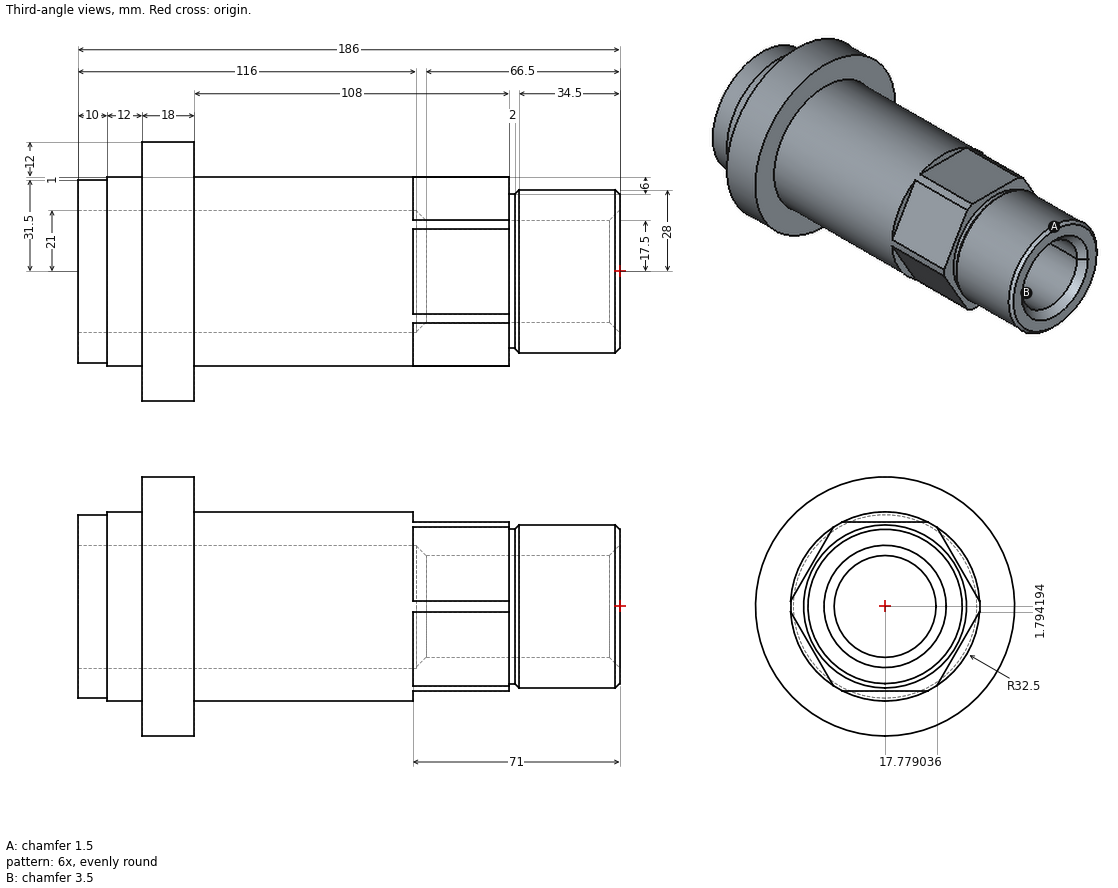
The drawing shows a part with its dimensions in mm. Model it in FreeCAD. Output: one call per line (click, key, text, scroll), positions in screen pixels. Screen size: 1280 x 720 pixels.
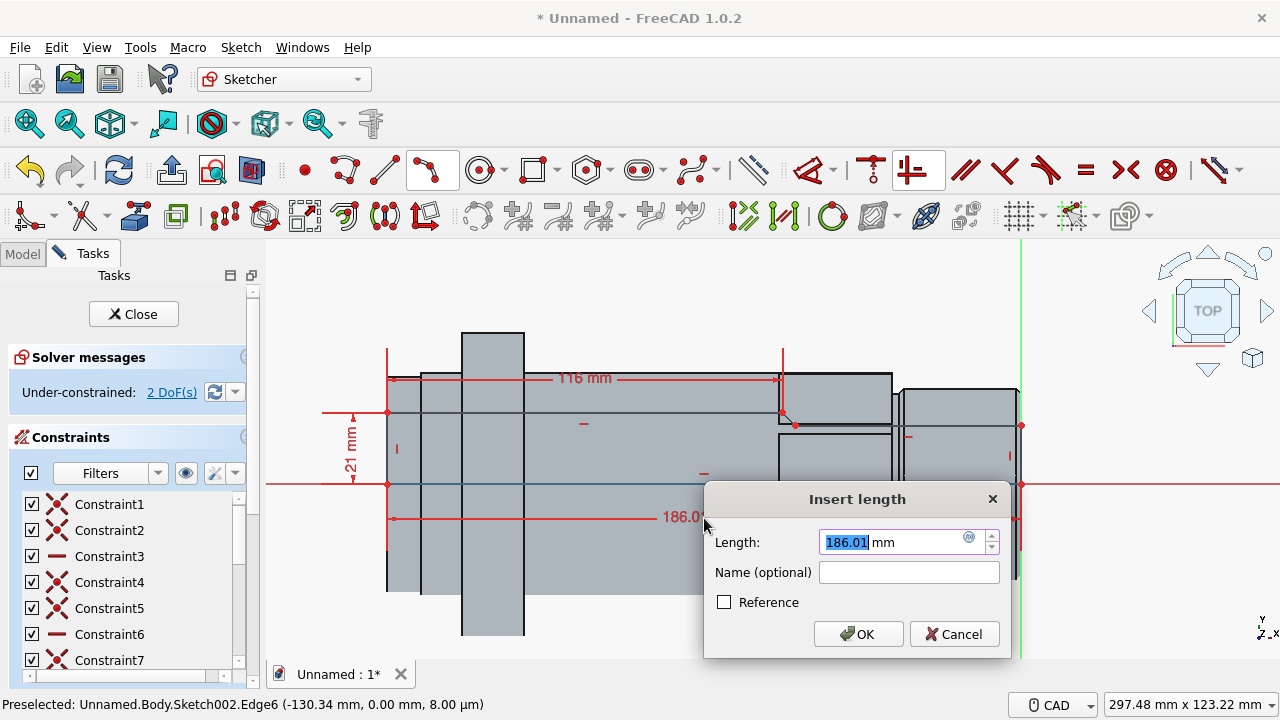
text(186)
key(Return)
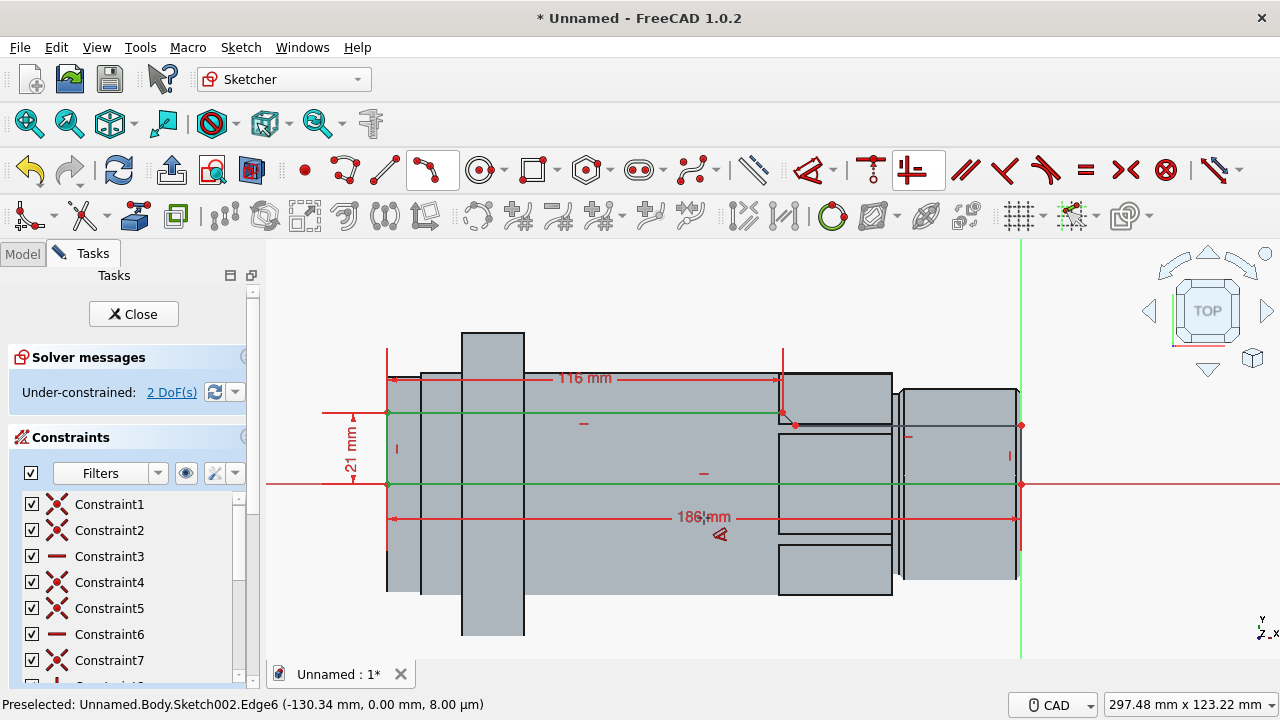
click(1021, 467)
click(1055, 455)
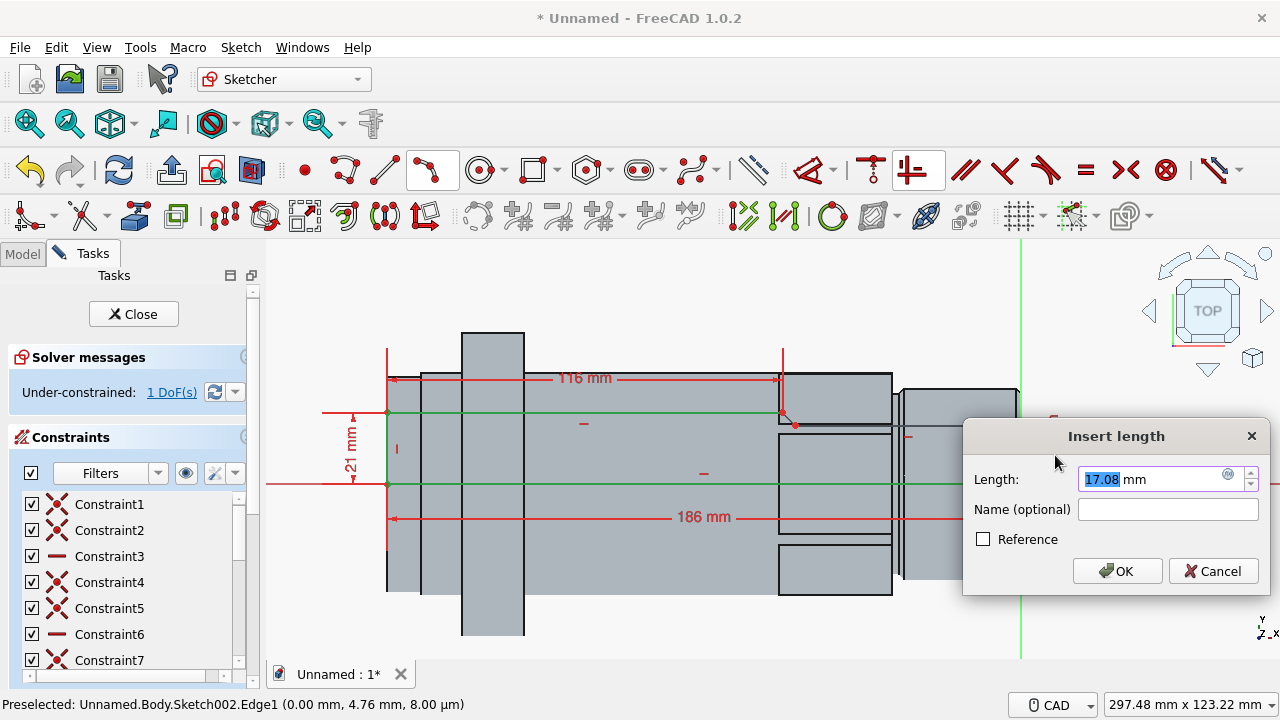
text(17.5)
key(Return)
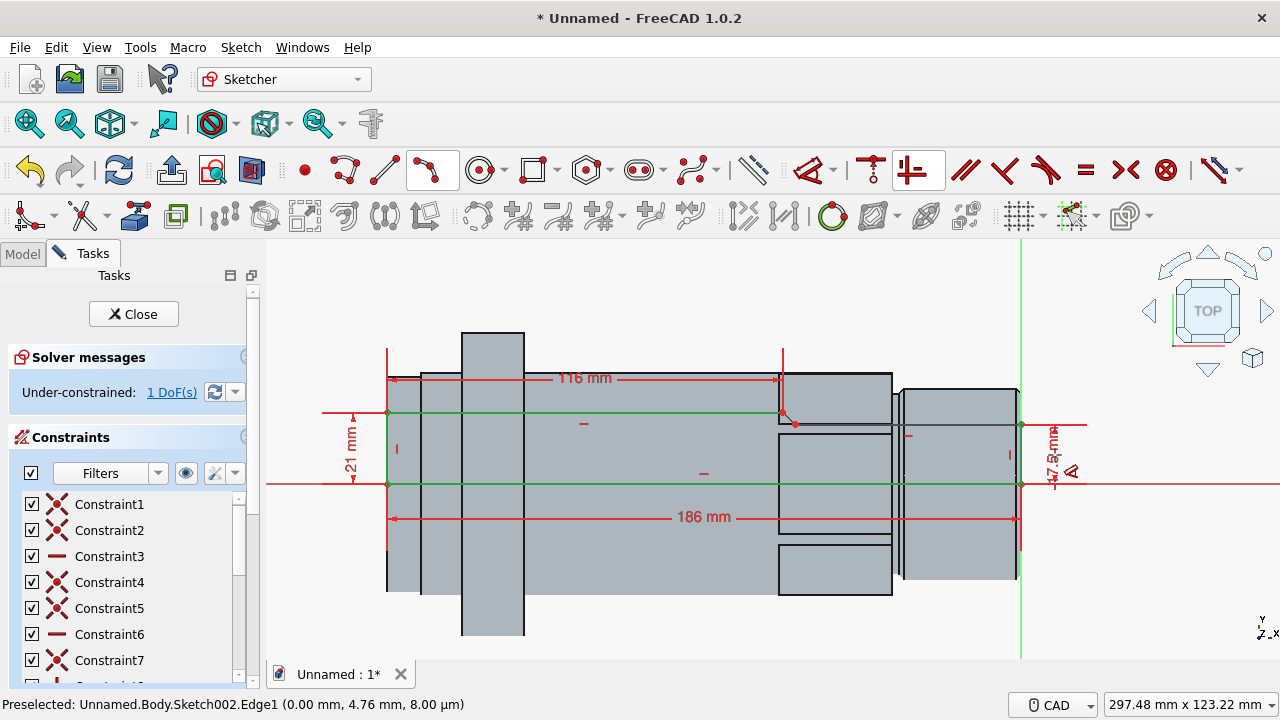
click(953, 425)
click(908, 391)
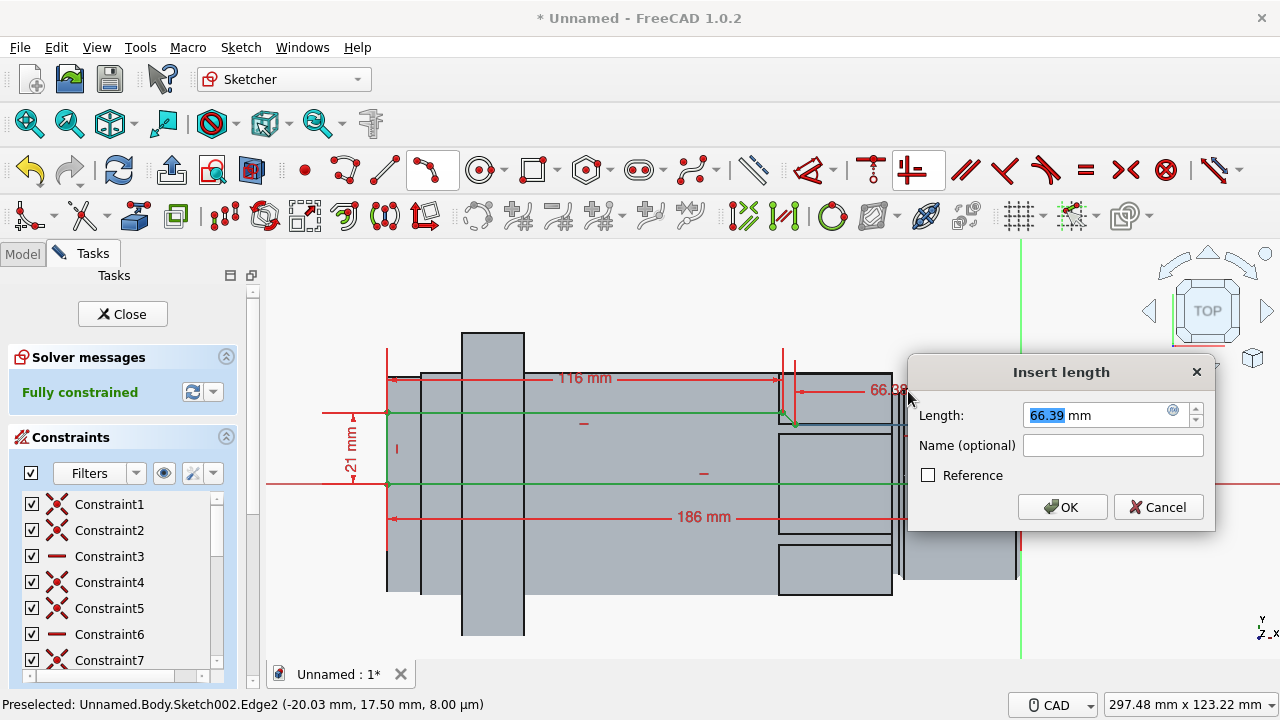
text(66.5)
key(Return)
key(Escape)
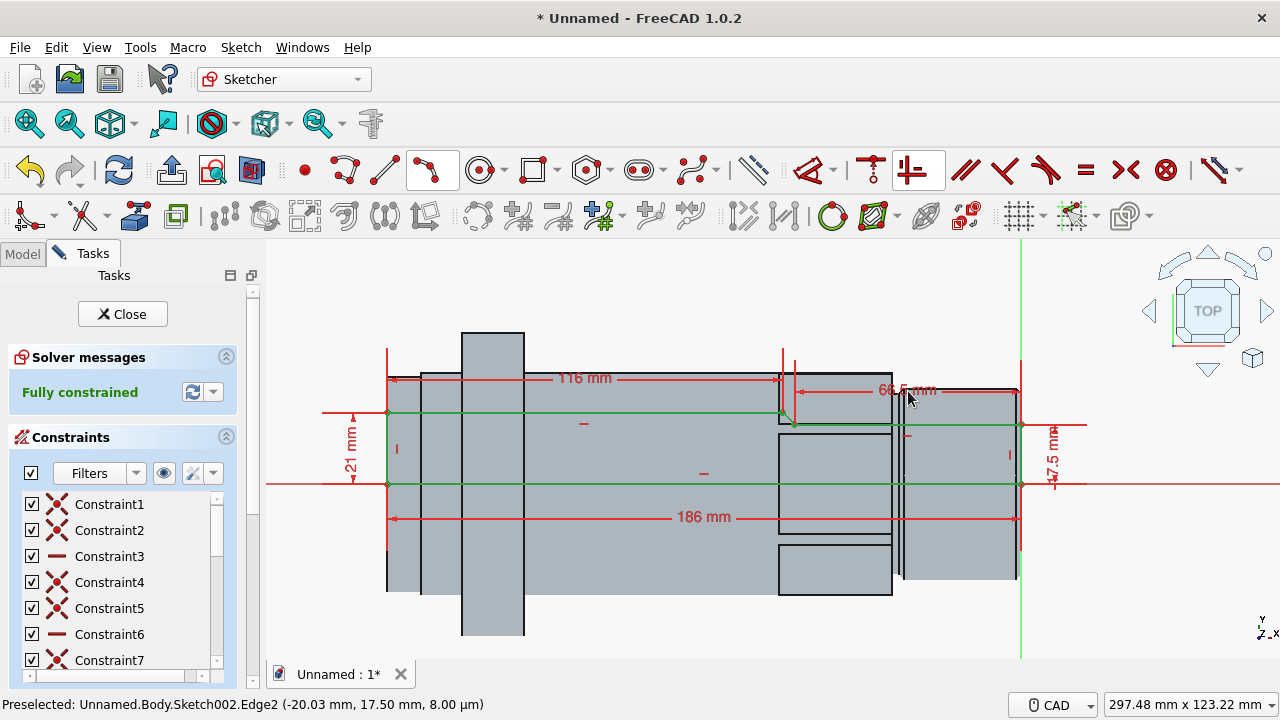
click(123, 314)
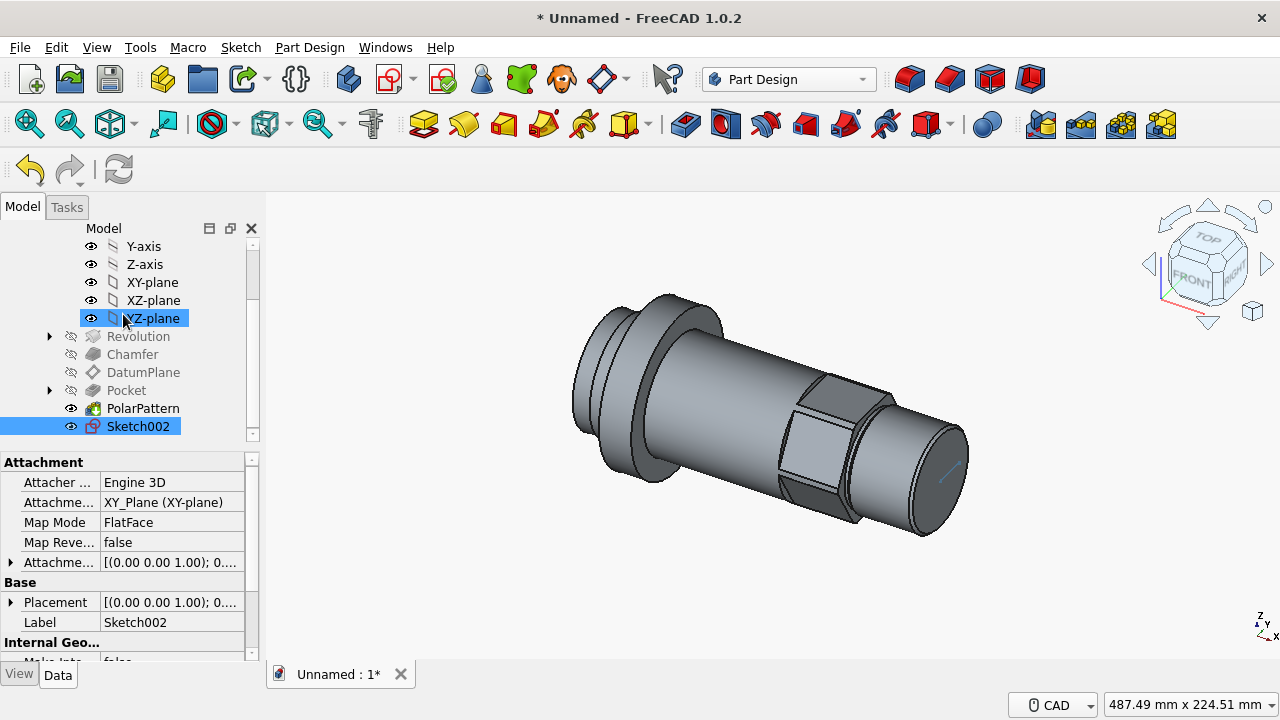
click(766, 124)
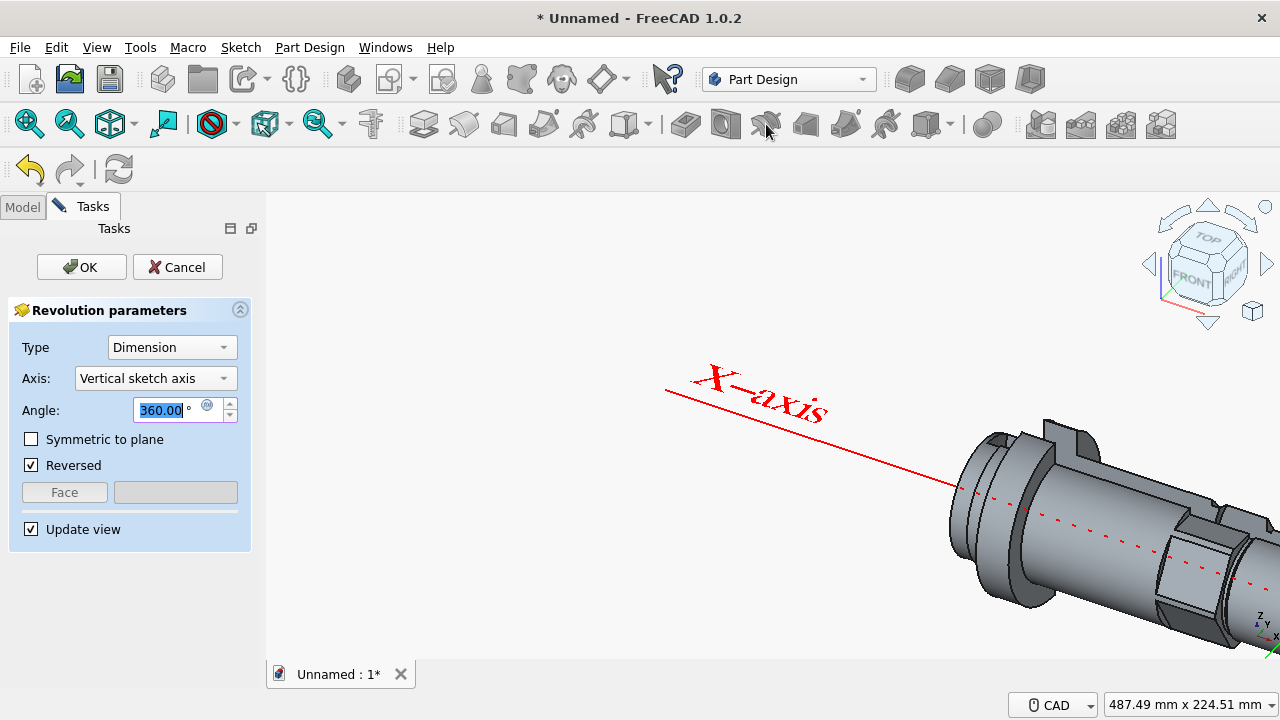
click(156, 378)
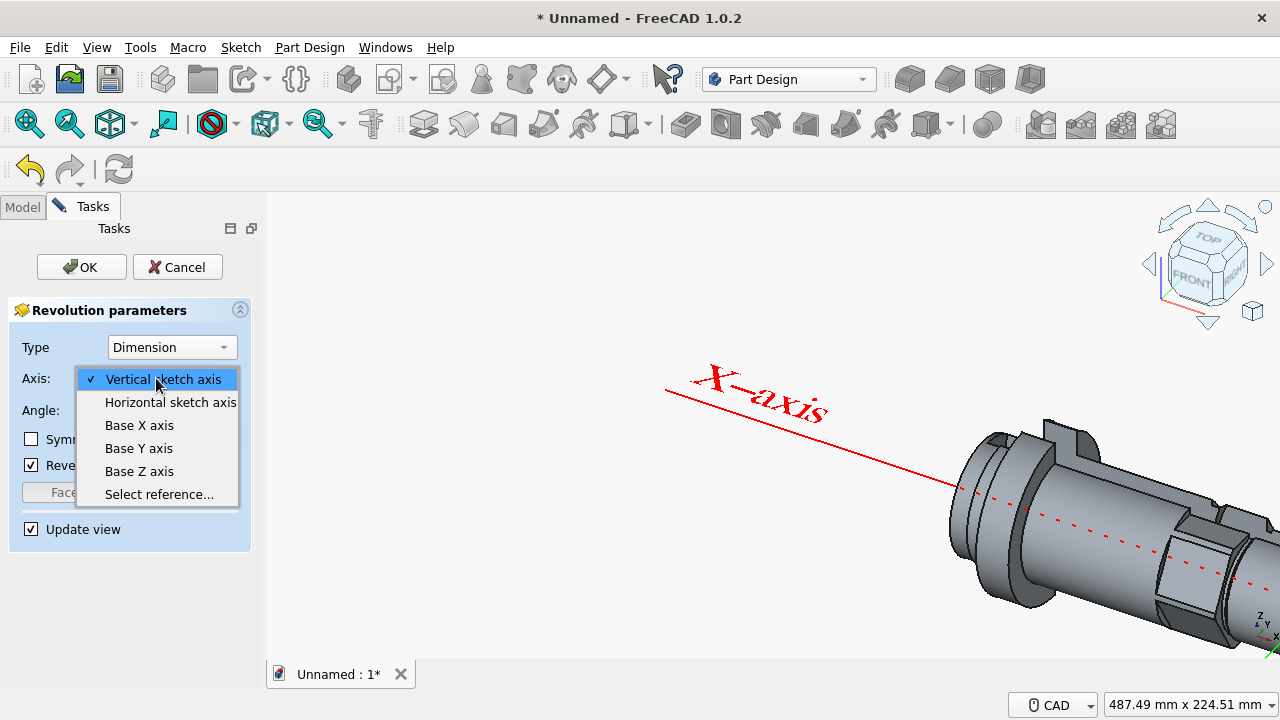
click(156, 402)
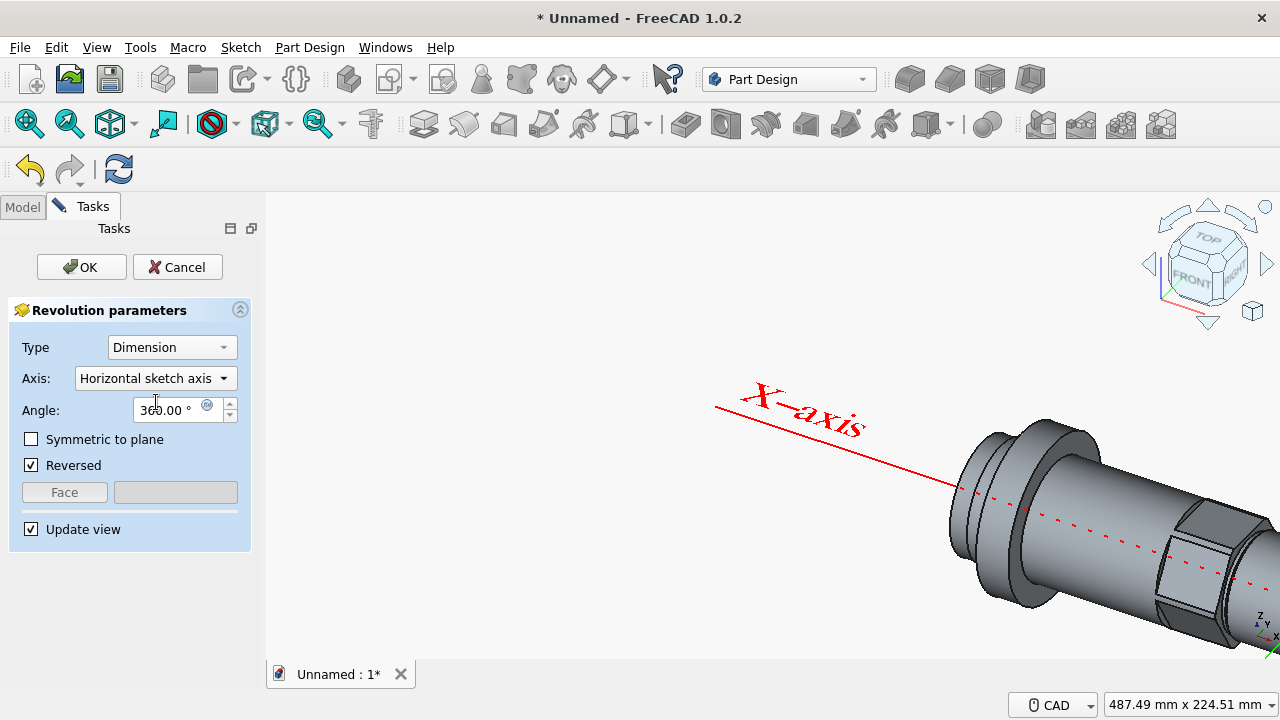
click(82, 267)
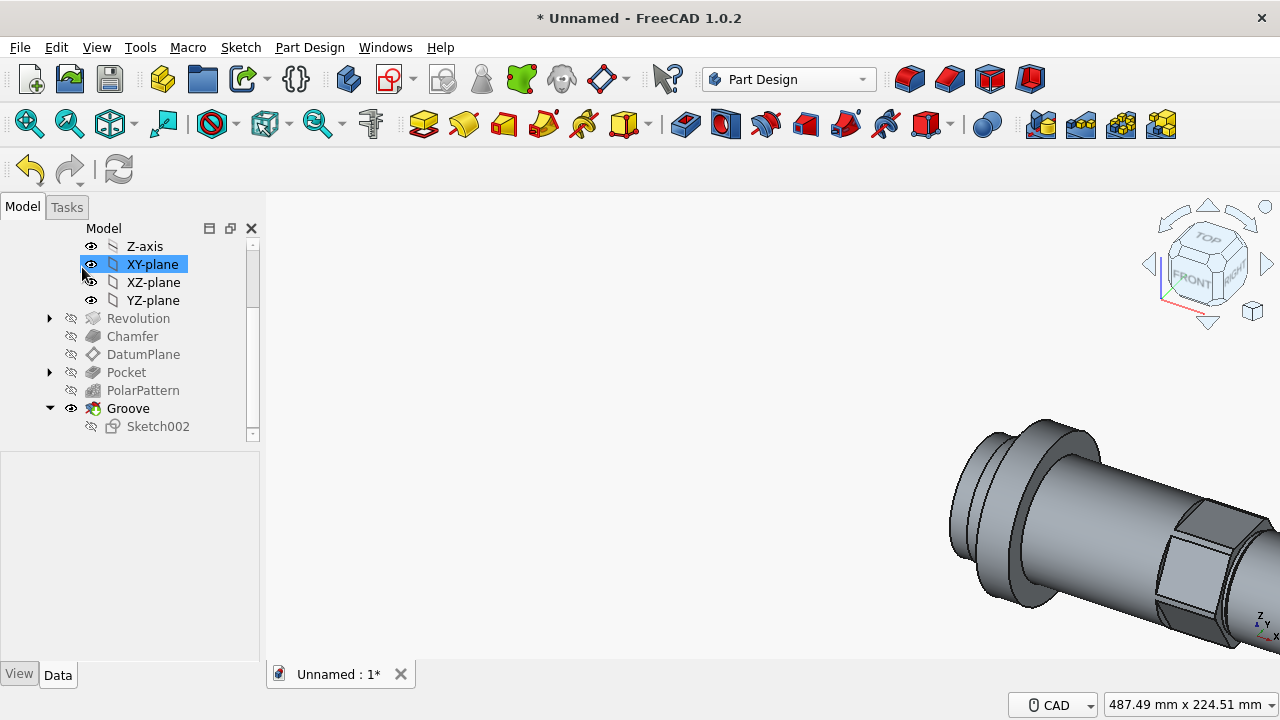
click(30, 124)